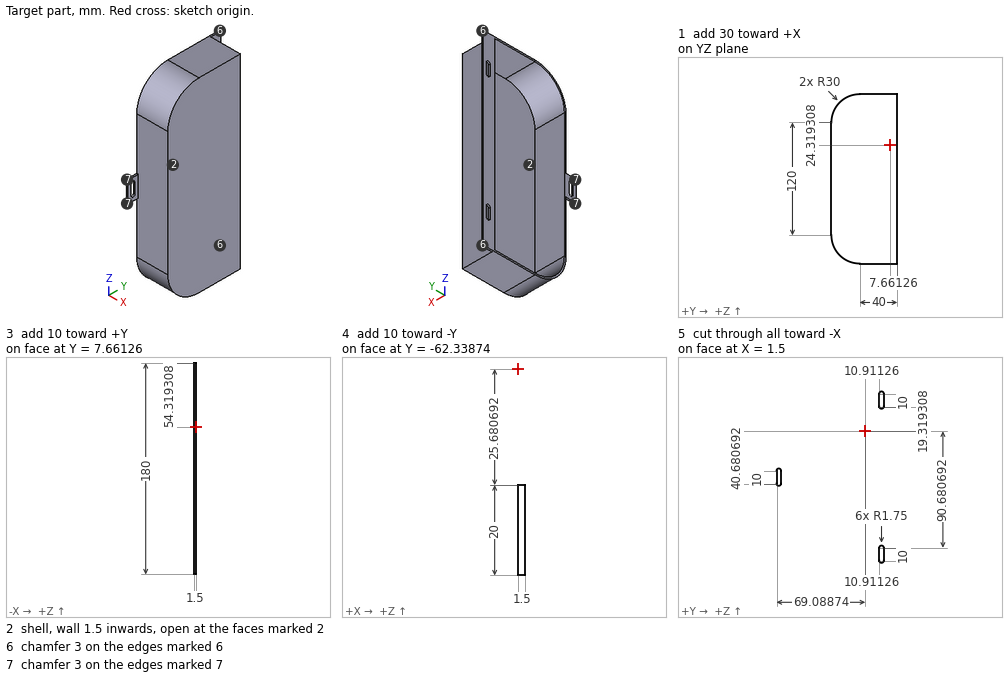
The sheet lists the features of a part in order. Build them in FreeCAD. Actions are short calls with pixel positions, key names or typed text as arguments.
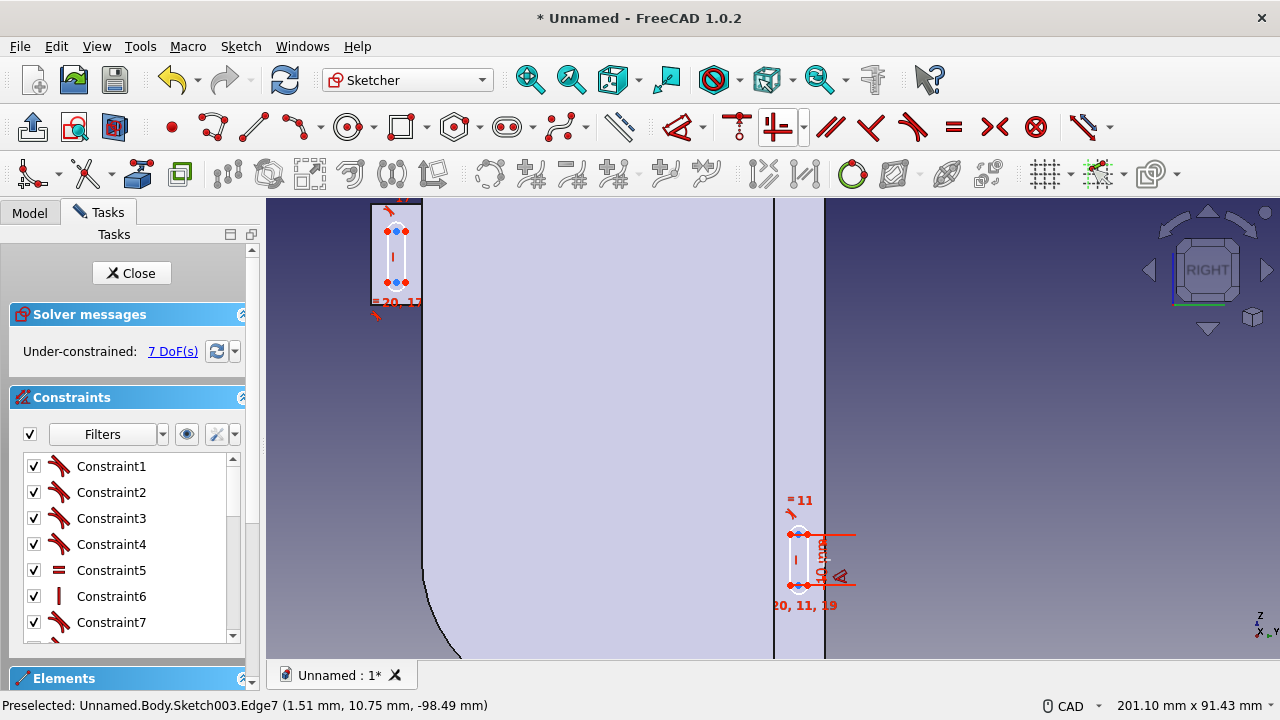
click(388, 267)
click(354, 257)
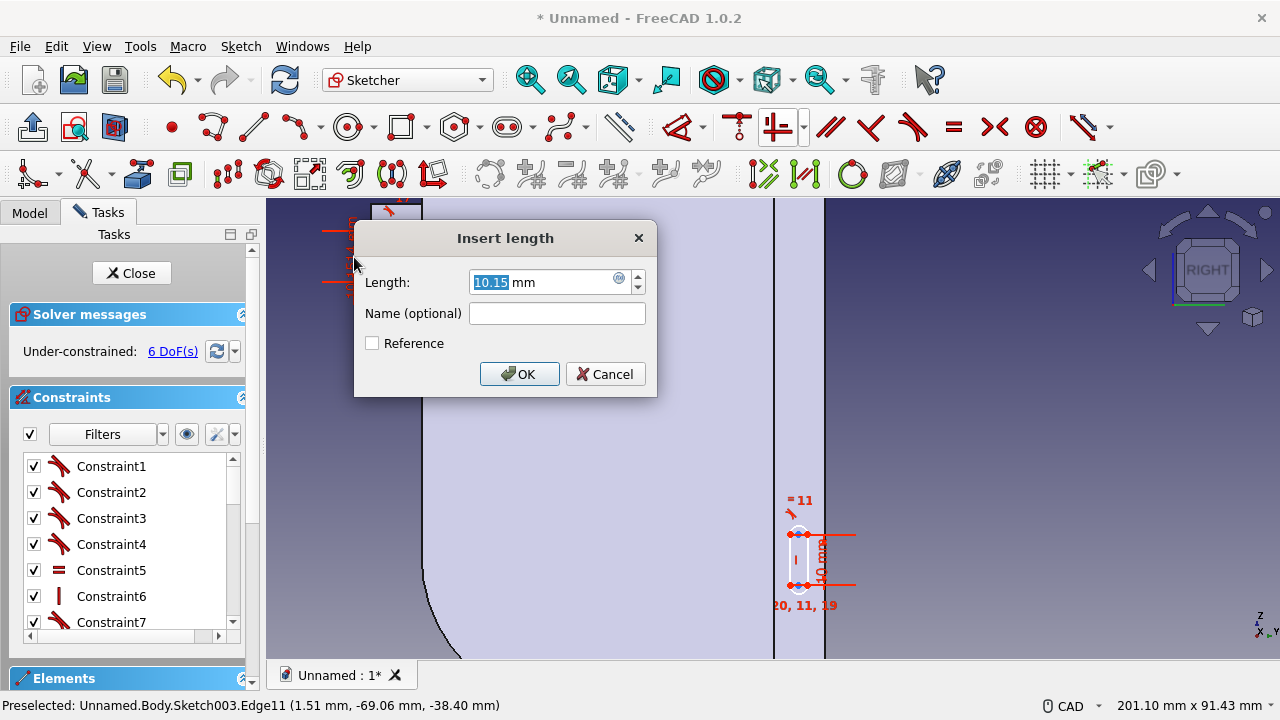
text(10)
key(Return)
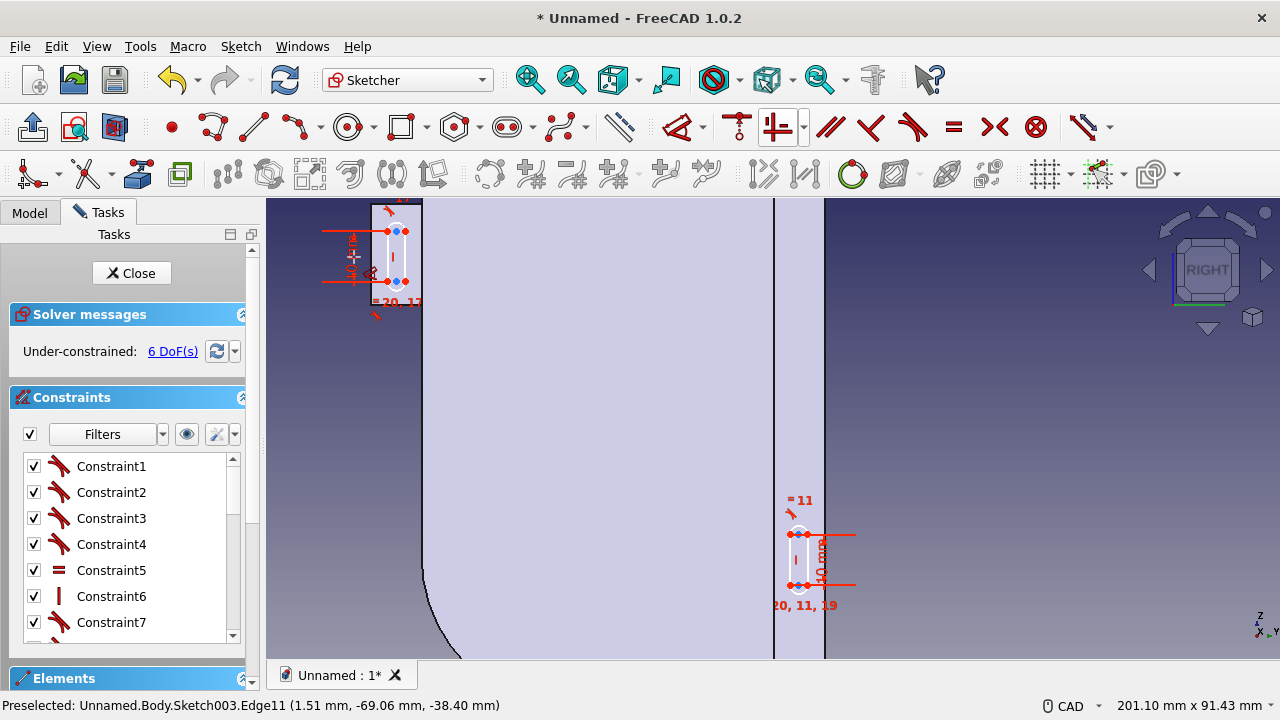
scroll(791, 571, down, 4)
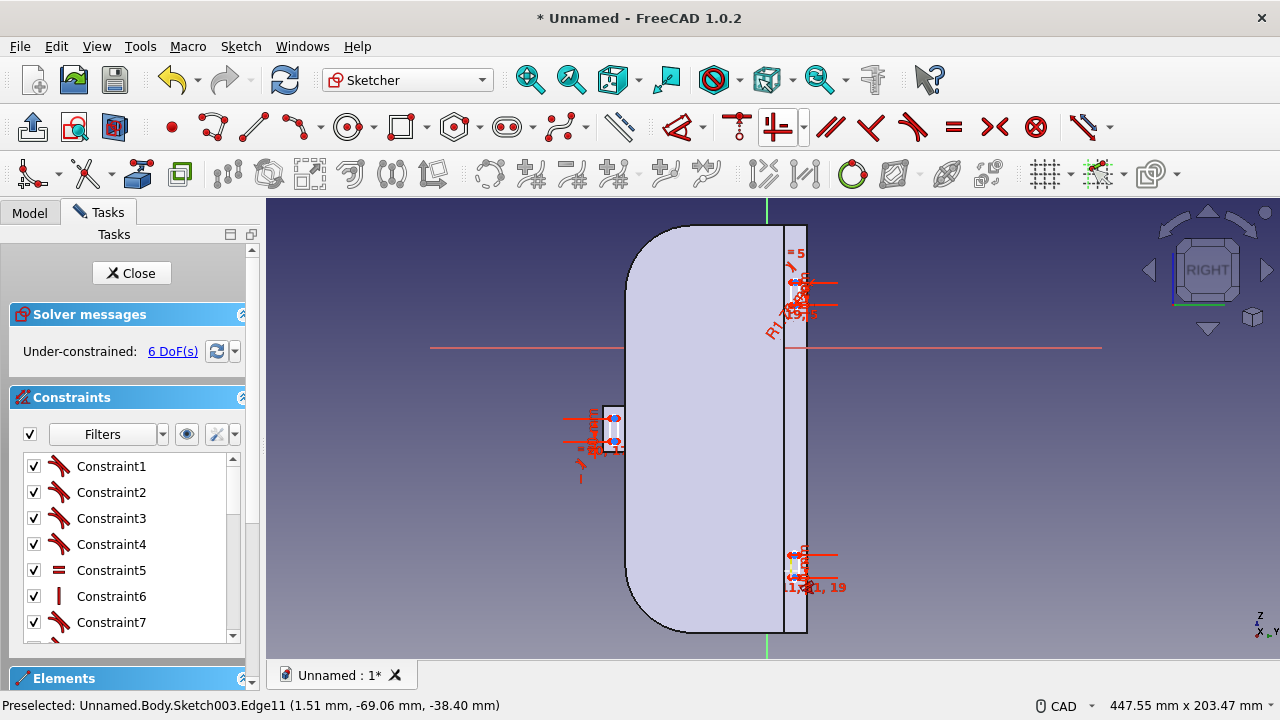
scroll(791, 305, up, 6)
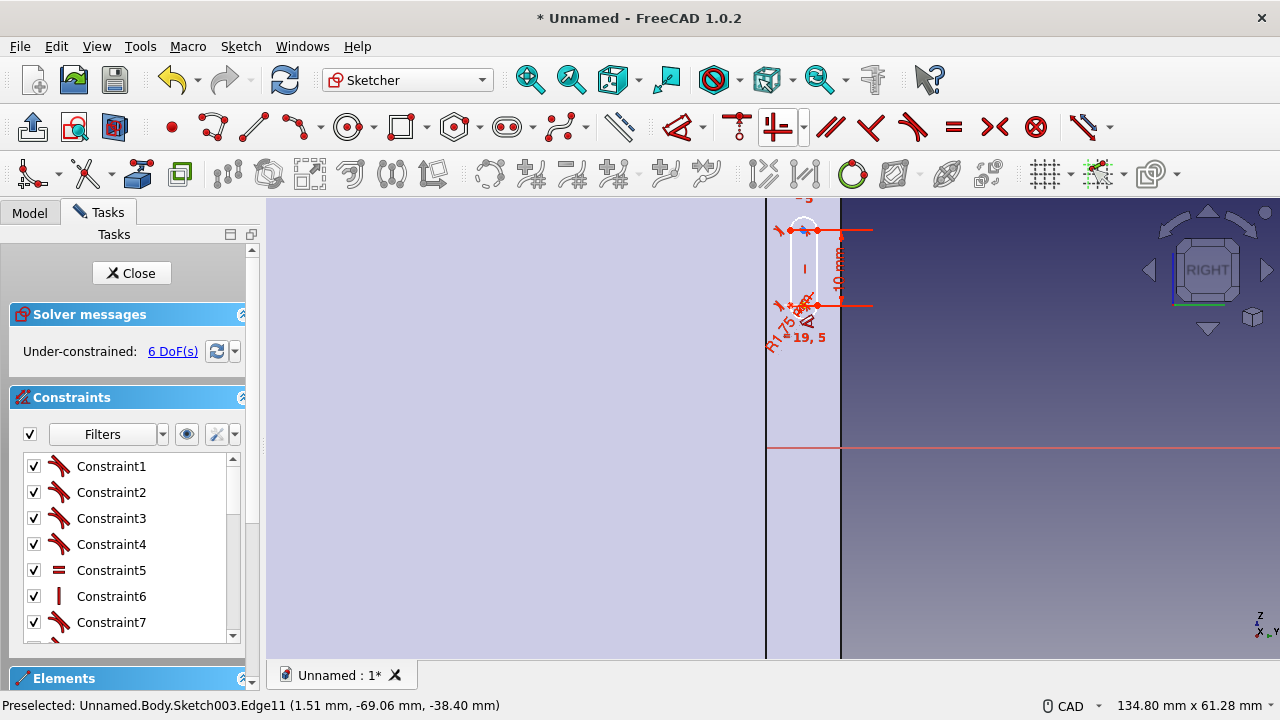
click(791, 306)
click(750, 272)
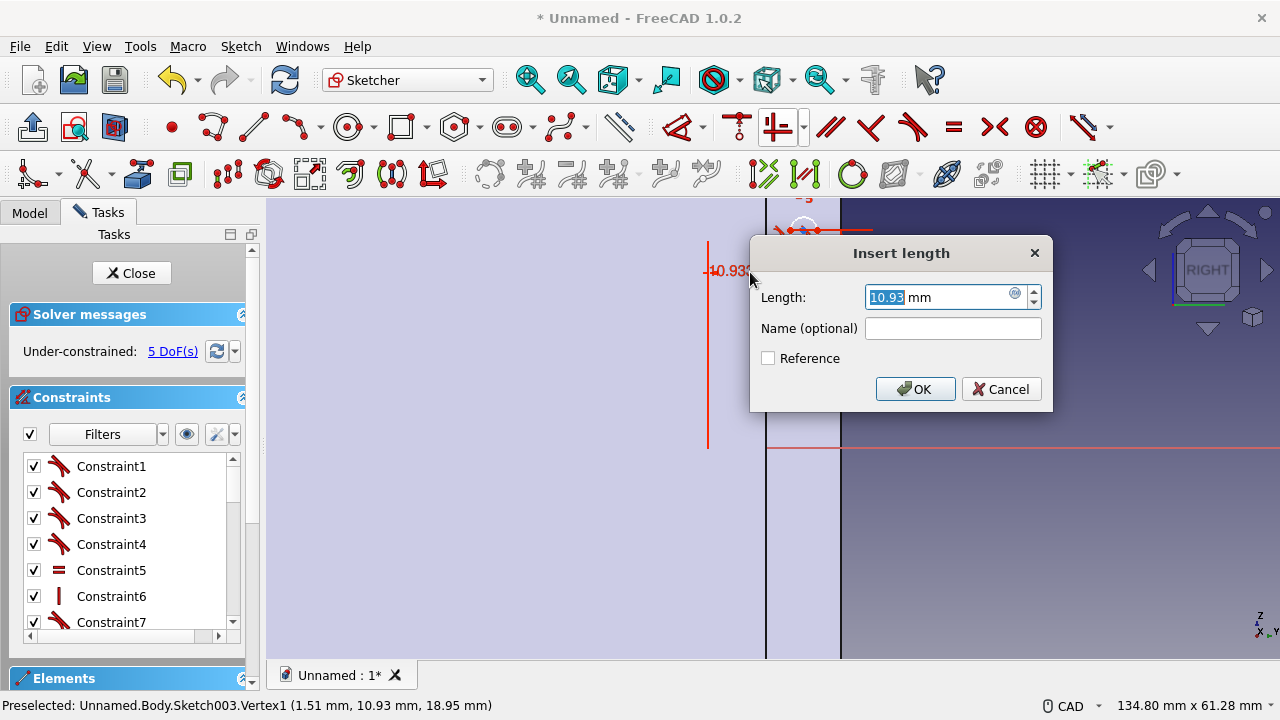
text(10.91126)
key(Return)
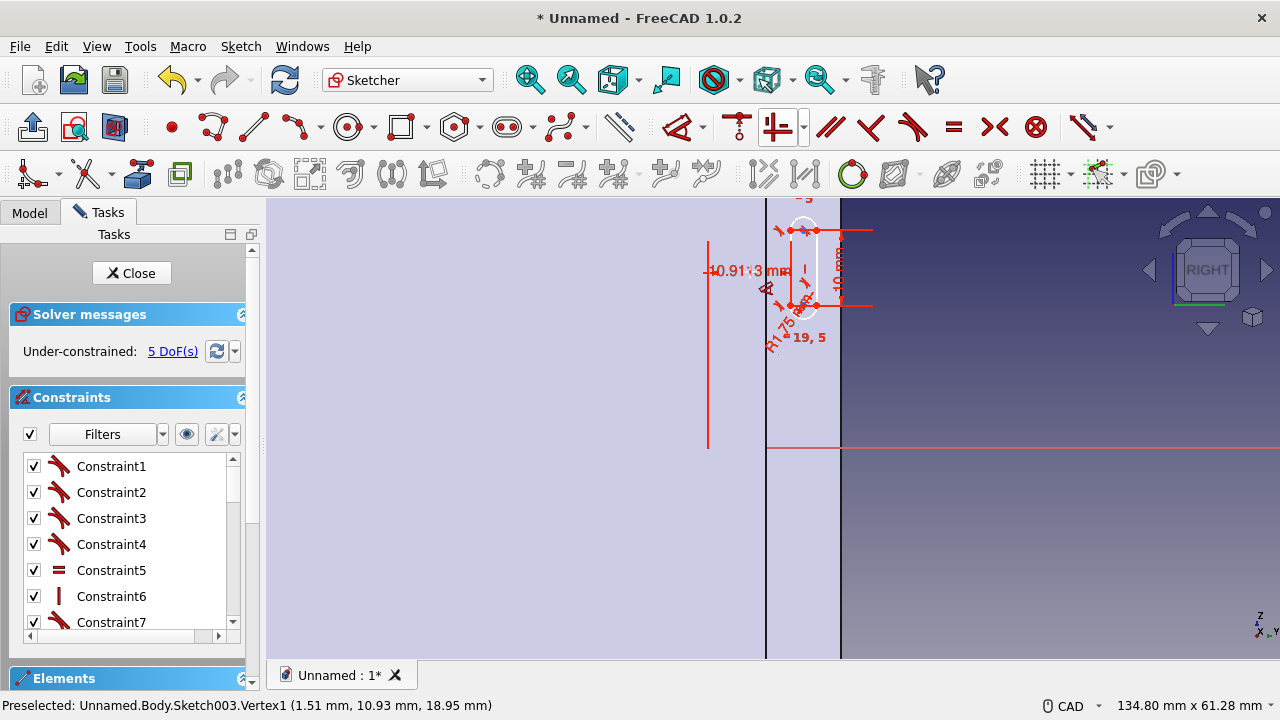
scroll(791, 304, down, 6)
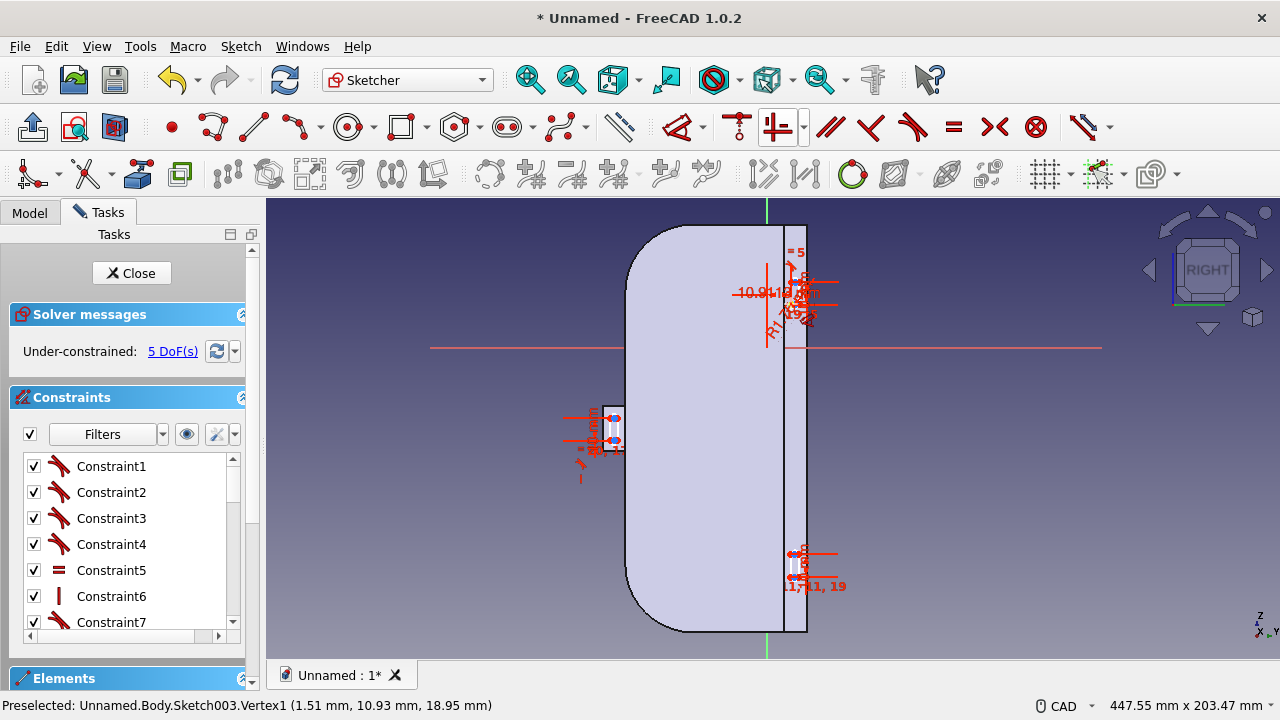
scroll(791, 577, up, 6)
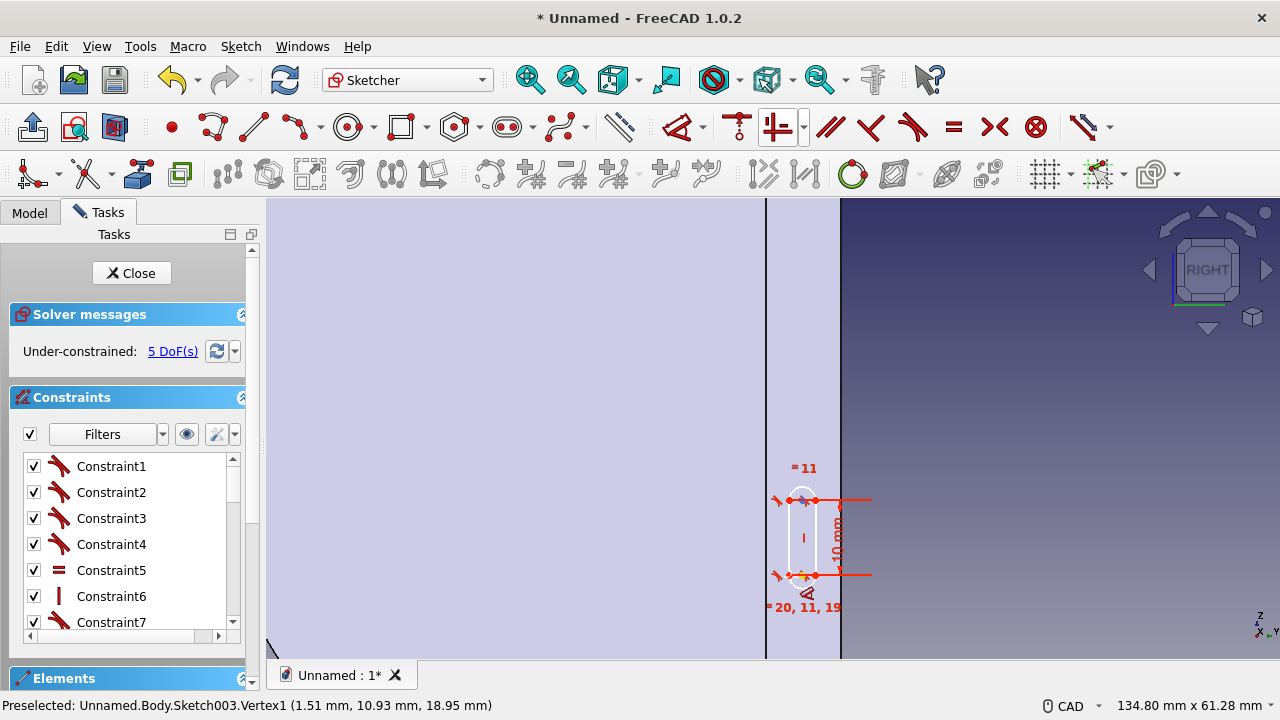
click(789, 575)
click(749, 609)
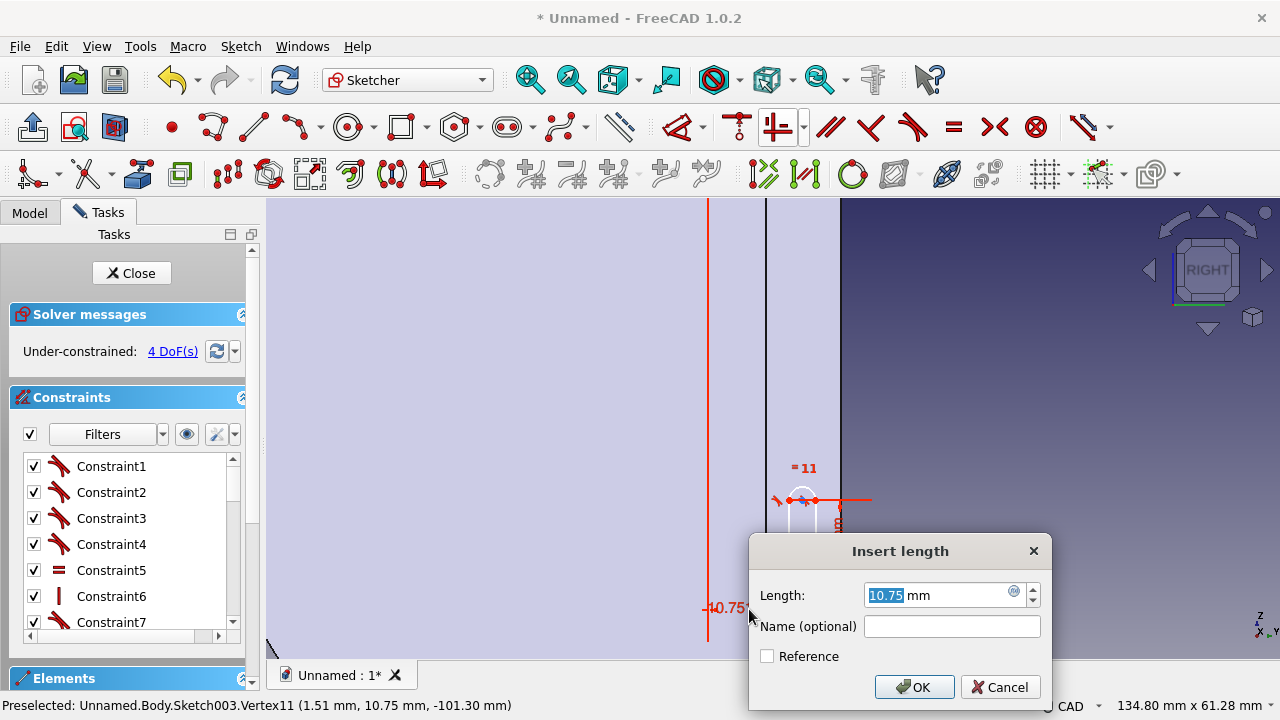
text(10.91126)
key(Return)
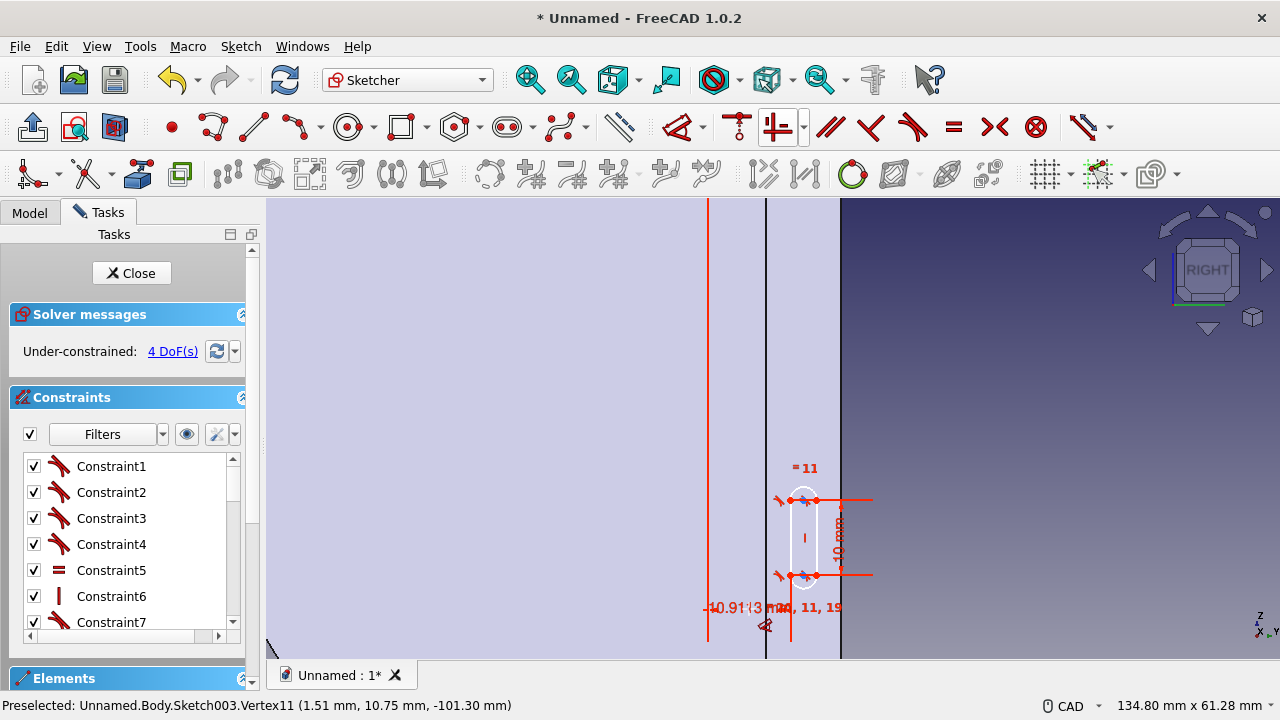
scroll(791, 578, down, 6)